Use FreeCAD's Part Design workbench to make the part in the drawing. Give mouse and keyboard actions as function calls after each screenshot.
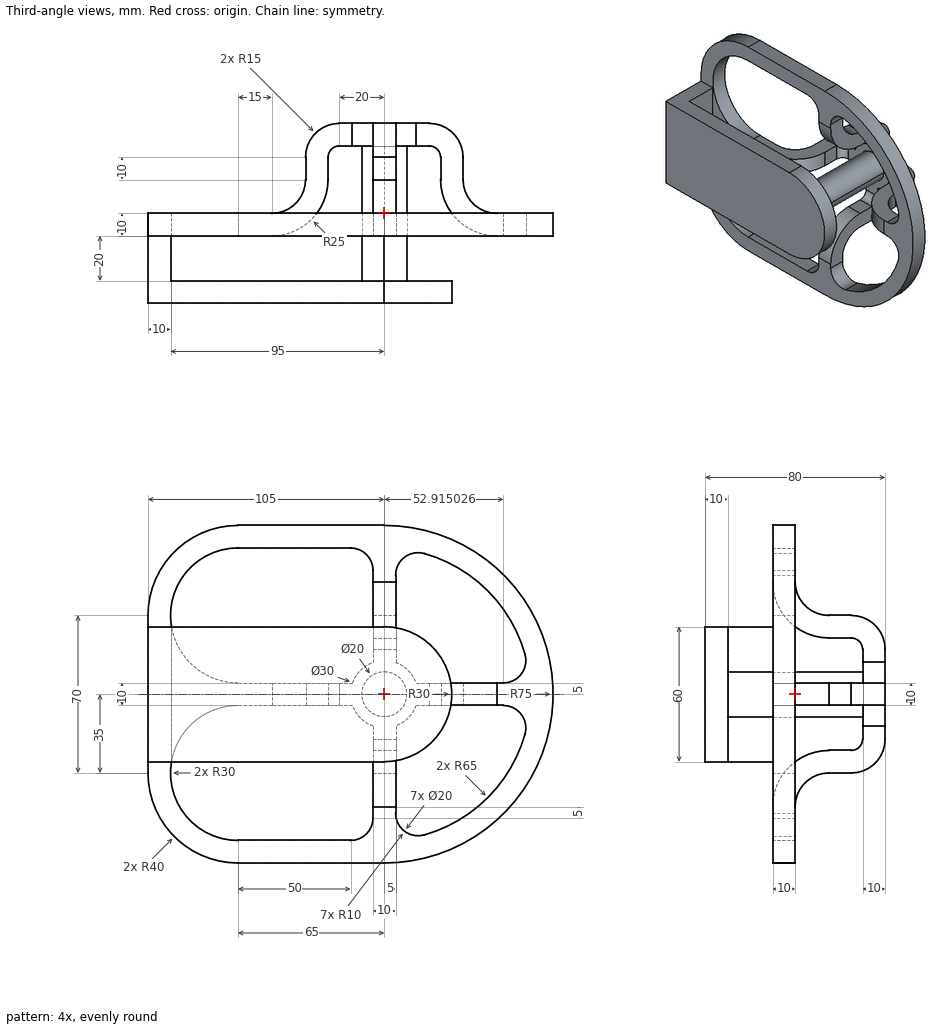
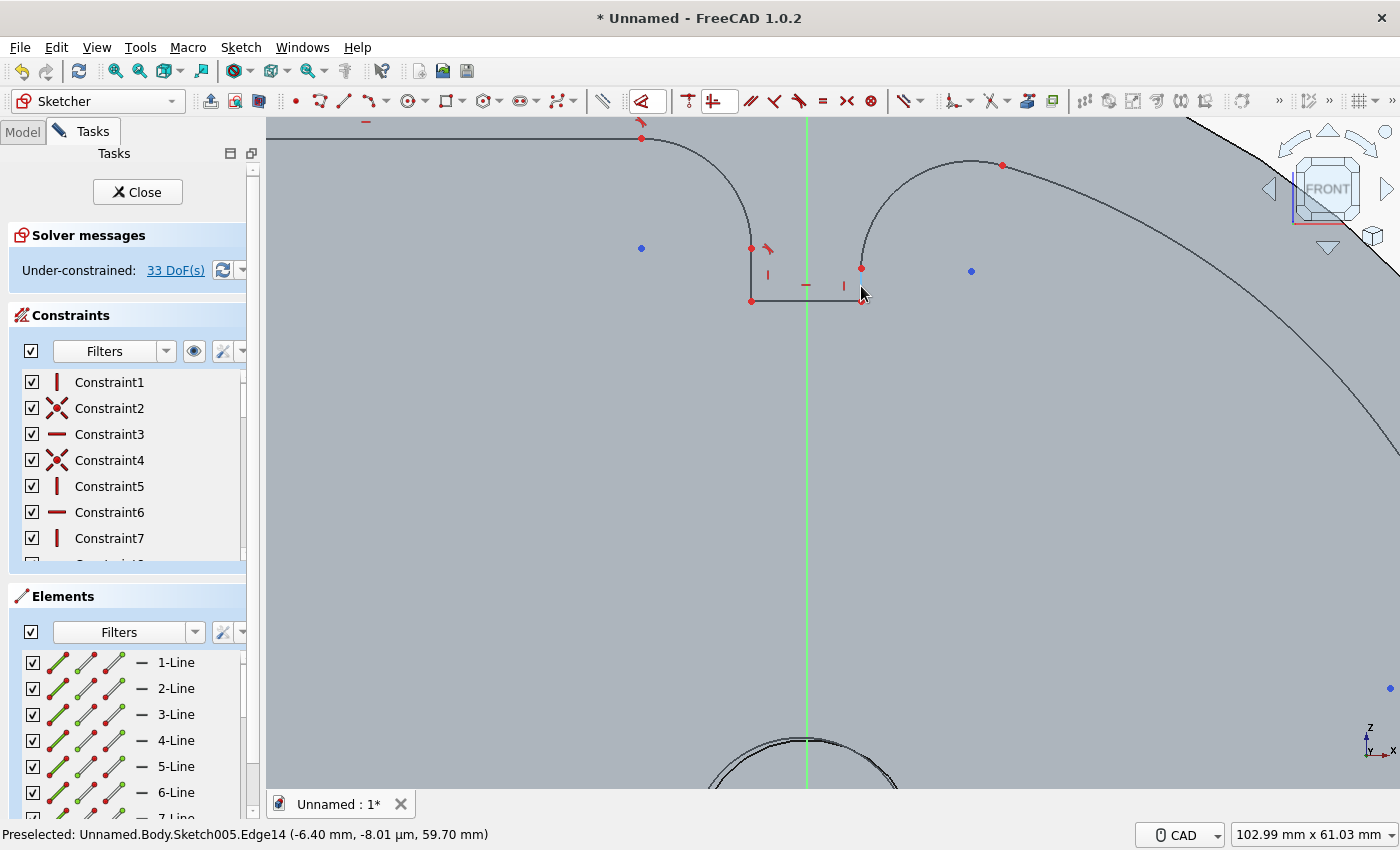
click(861, 285)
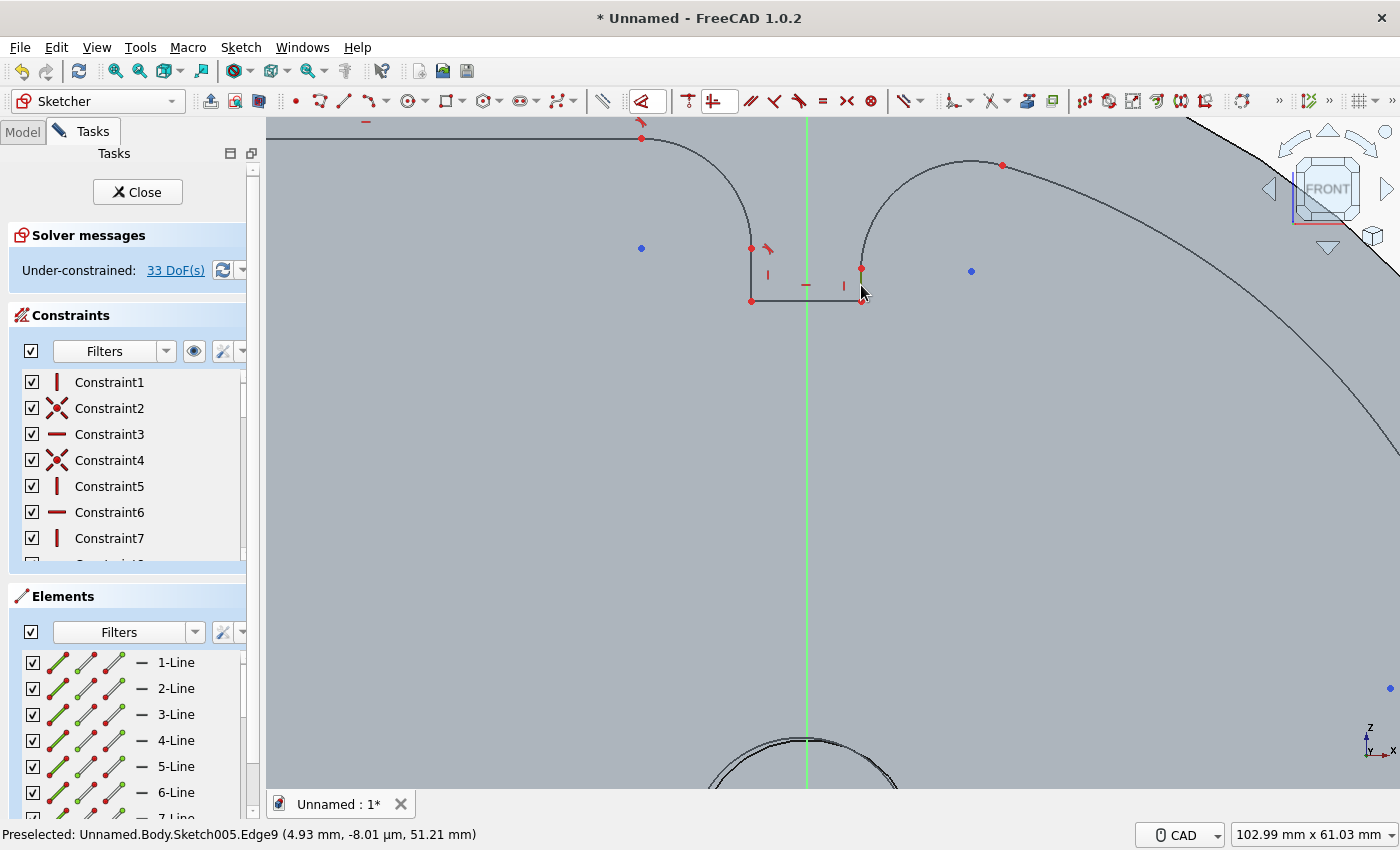
scroll(823, 282, down, 6)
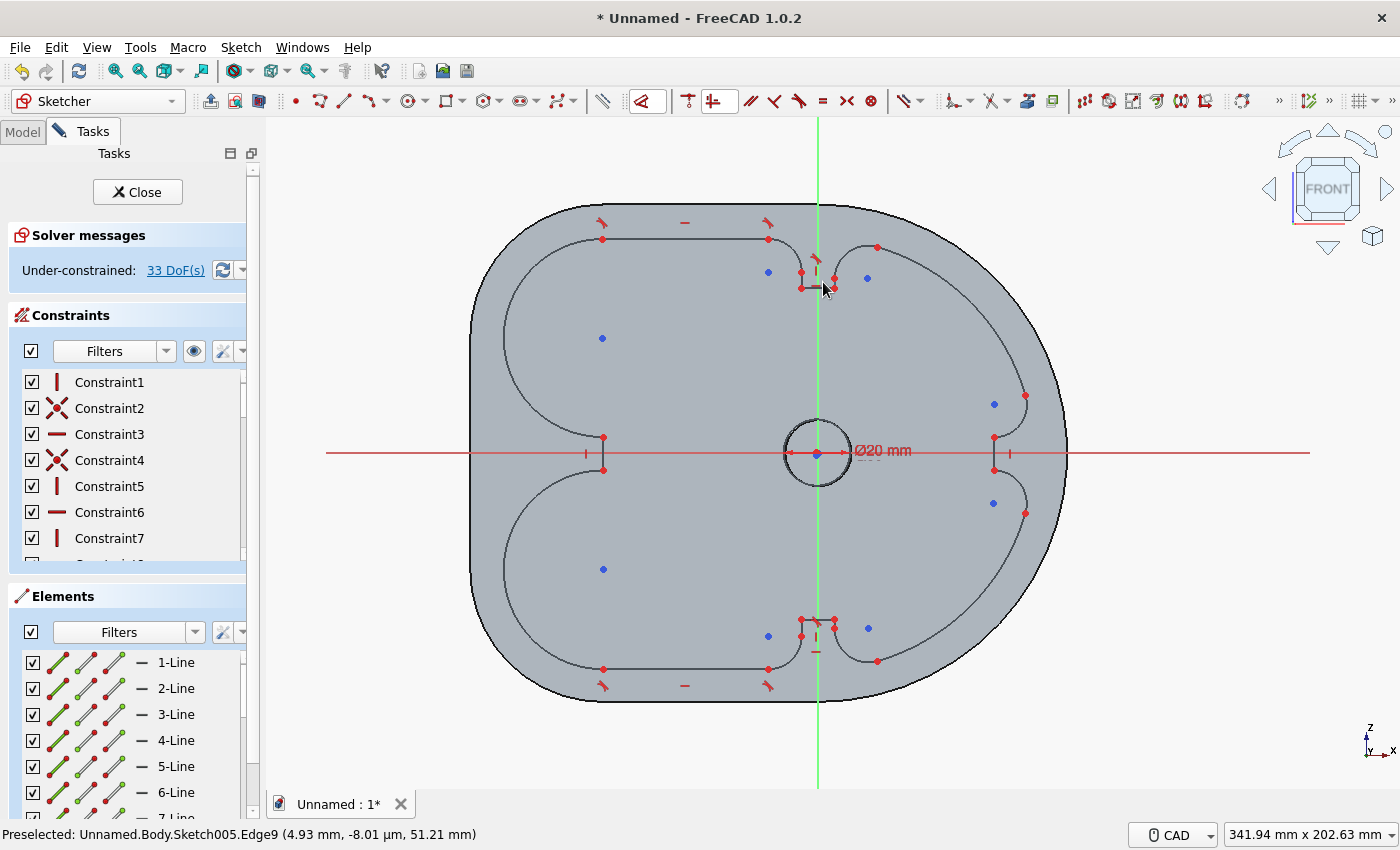
click(859, 247)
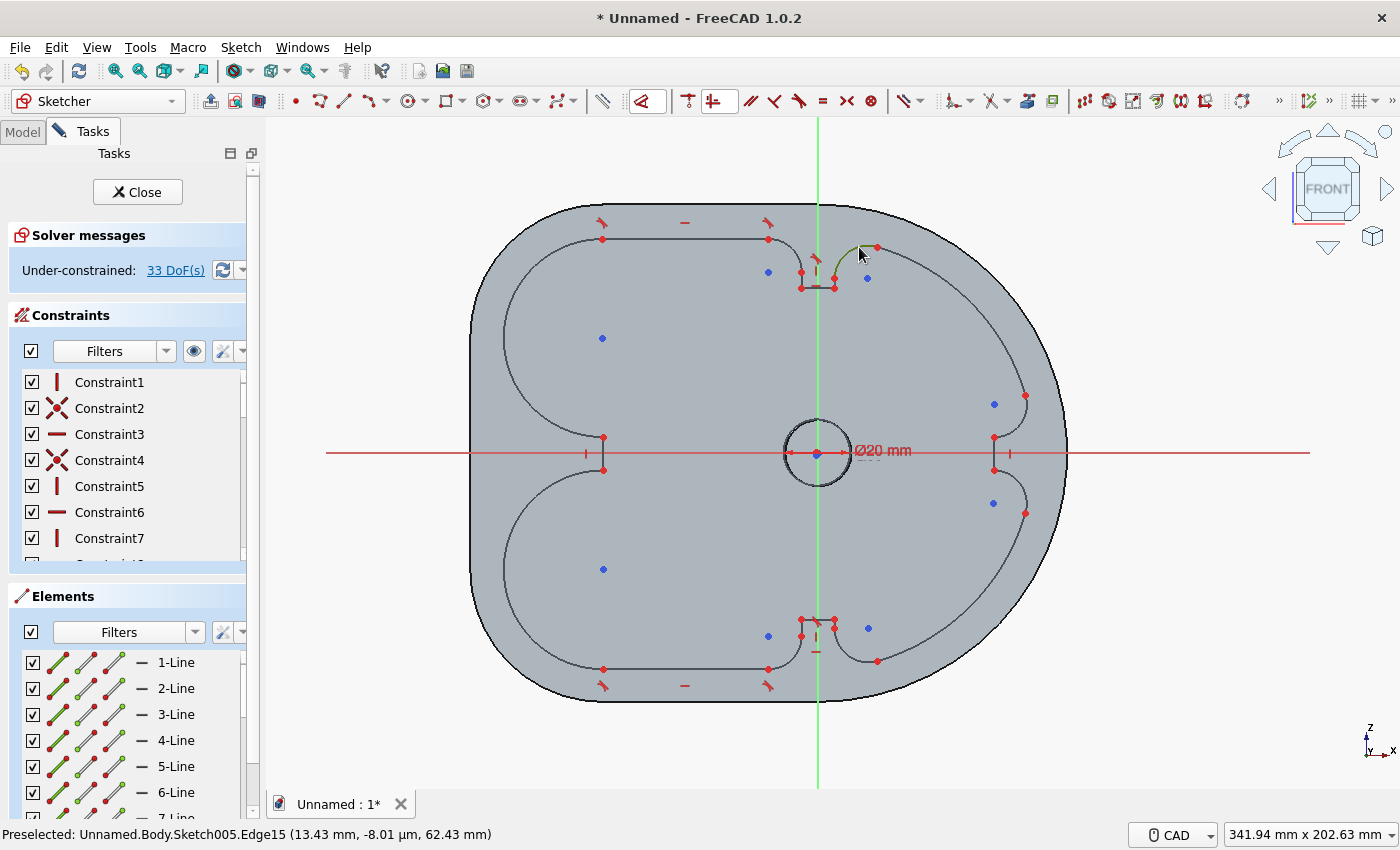
click(800, 102)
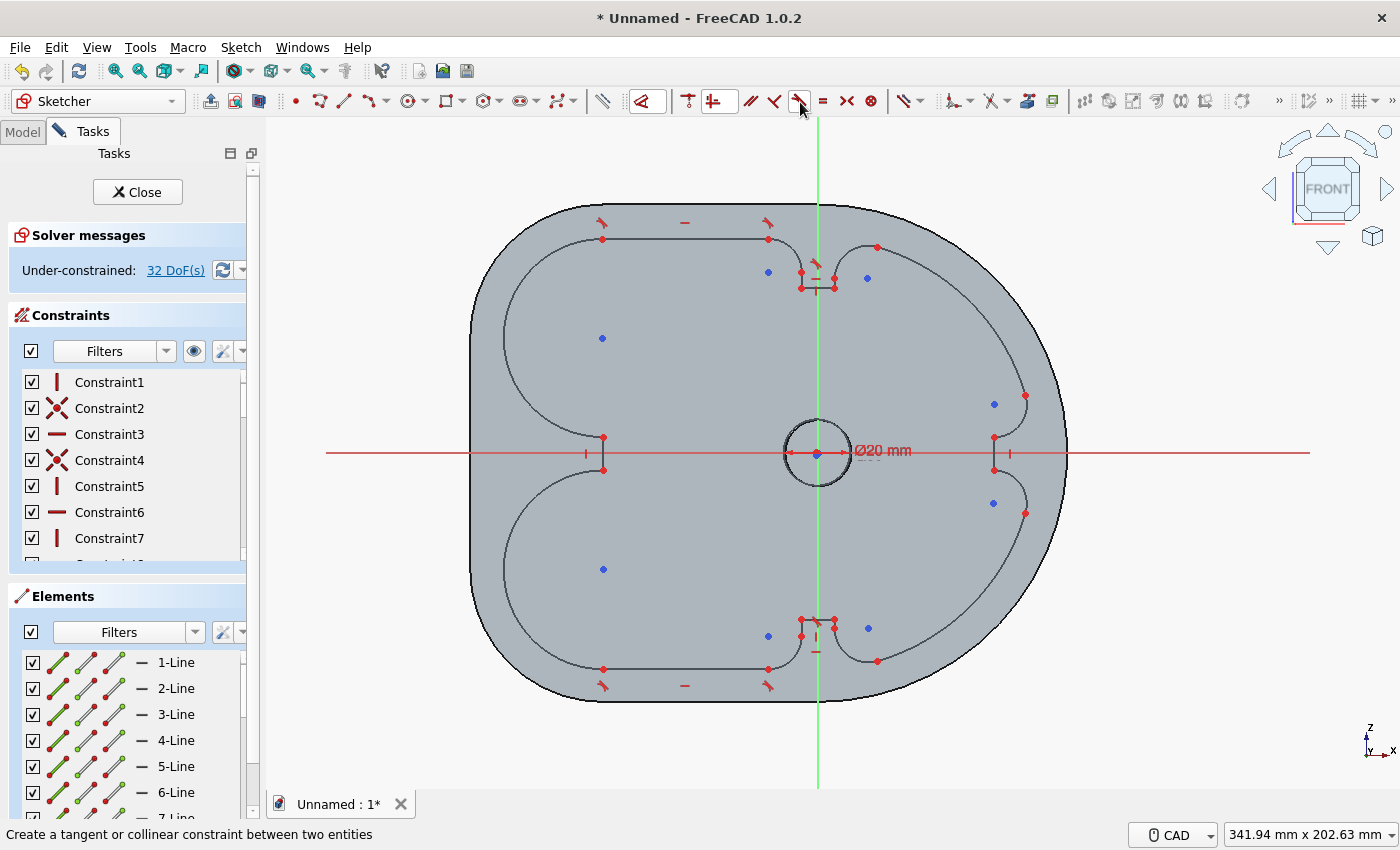
click(859, 247)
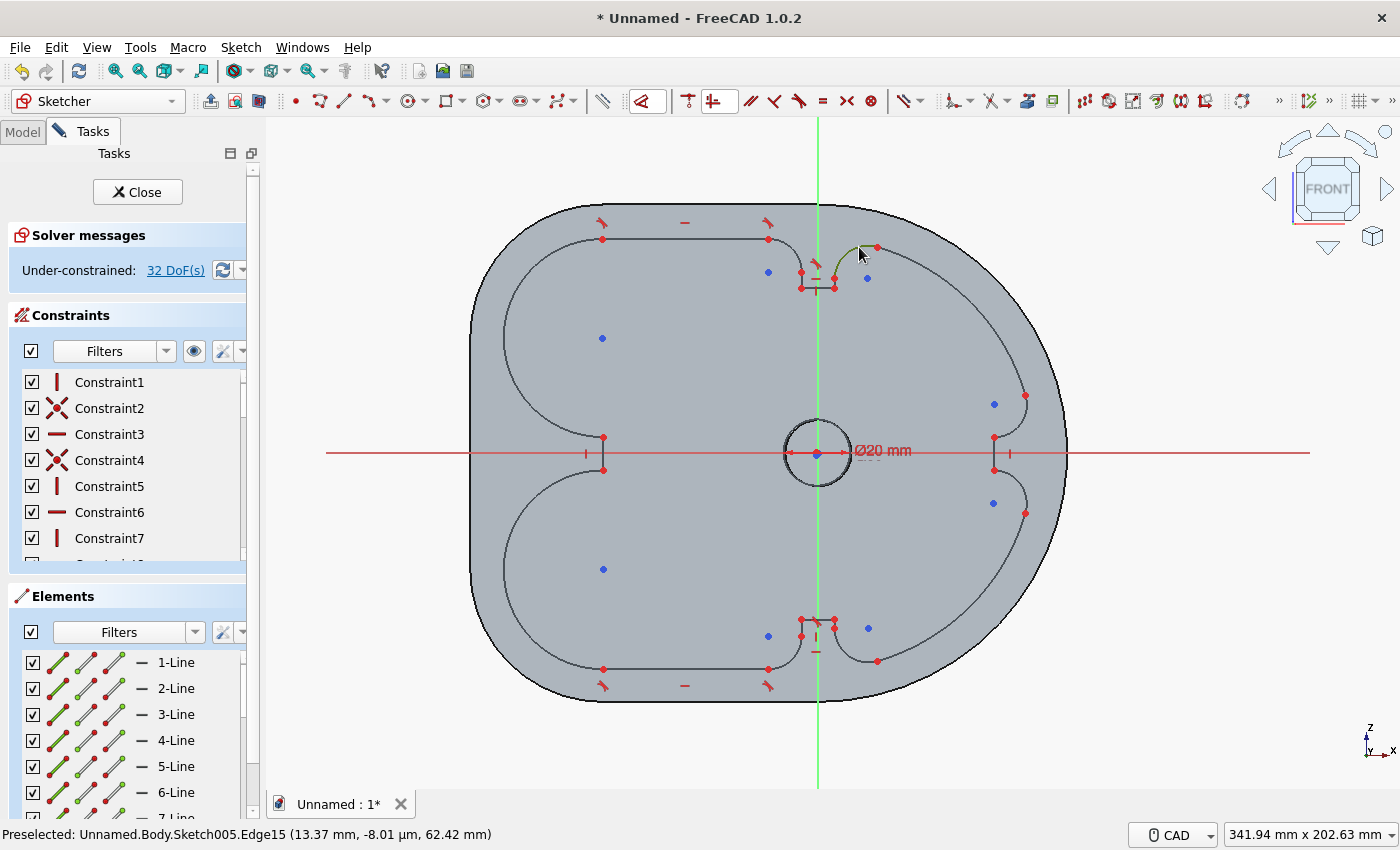
click(998, 336)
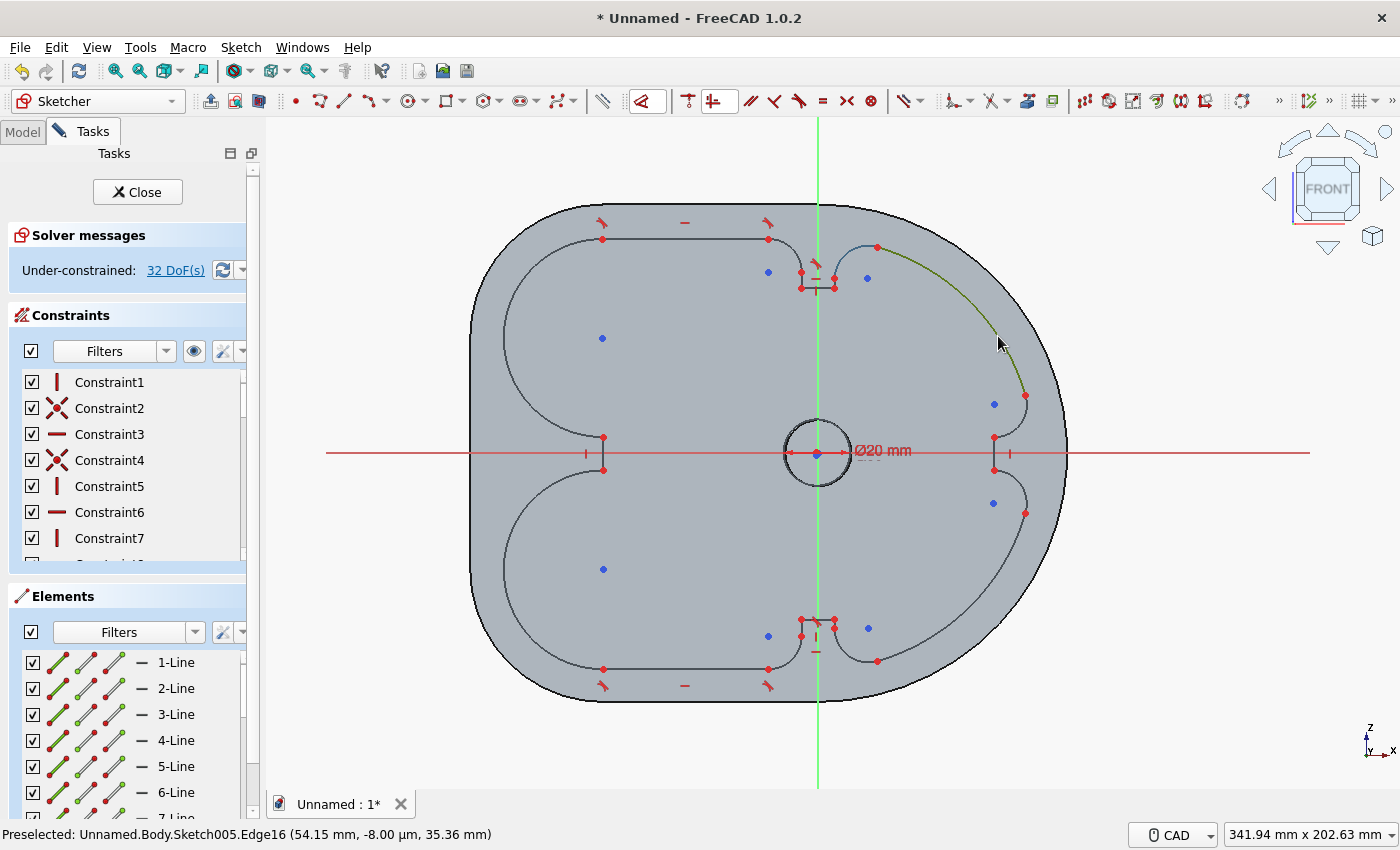
click(800, 102)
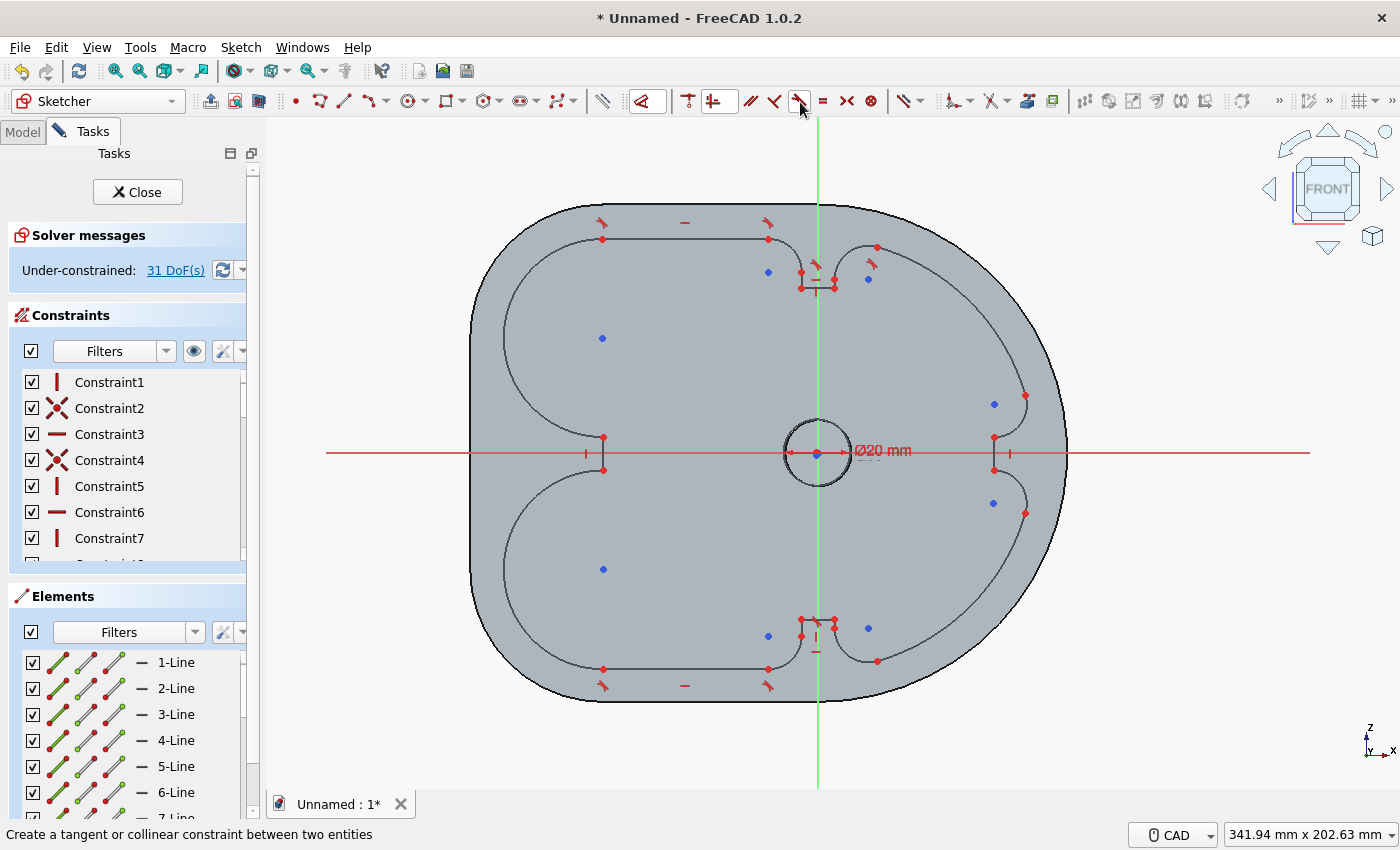
click(998, 336)